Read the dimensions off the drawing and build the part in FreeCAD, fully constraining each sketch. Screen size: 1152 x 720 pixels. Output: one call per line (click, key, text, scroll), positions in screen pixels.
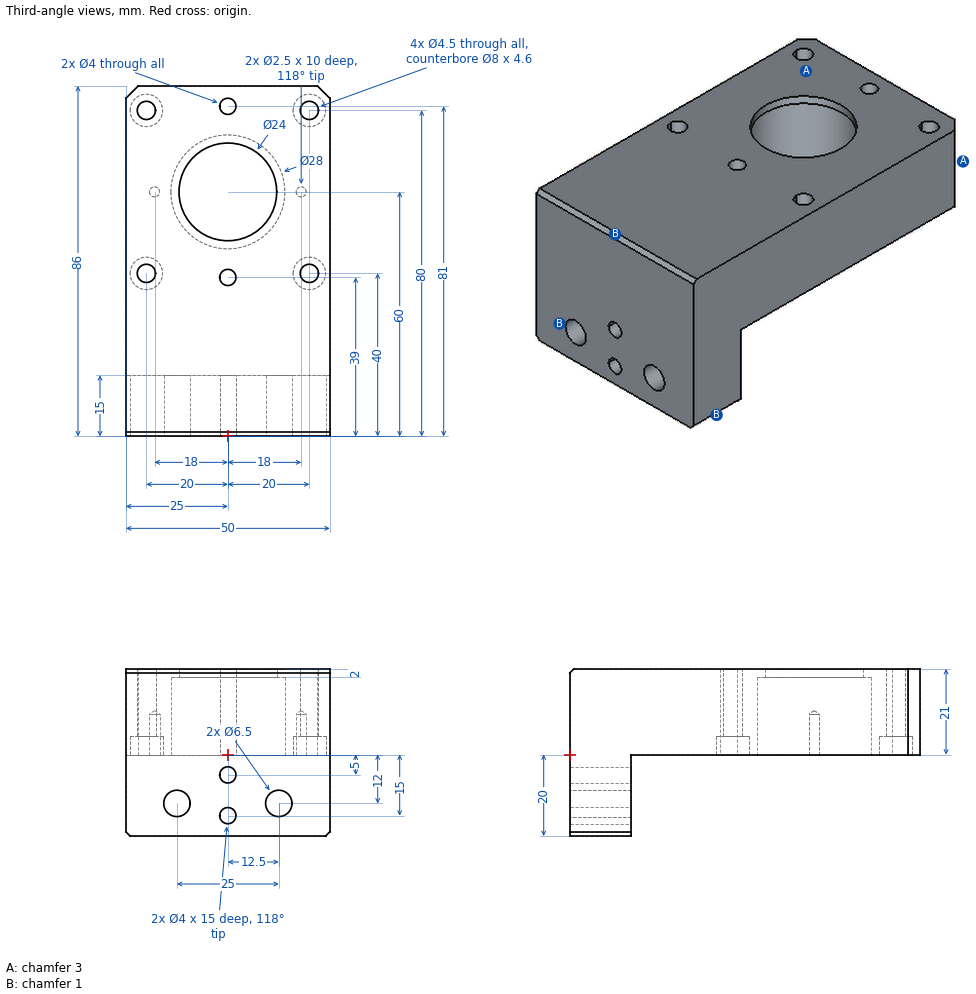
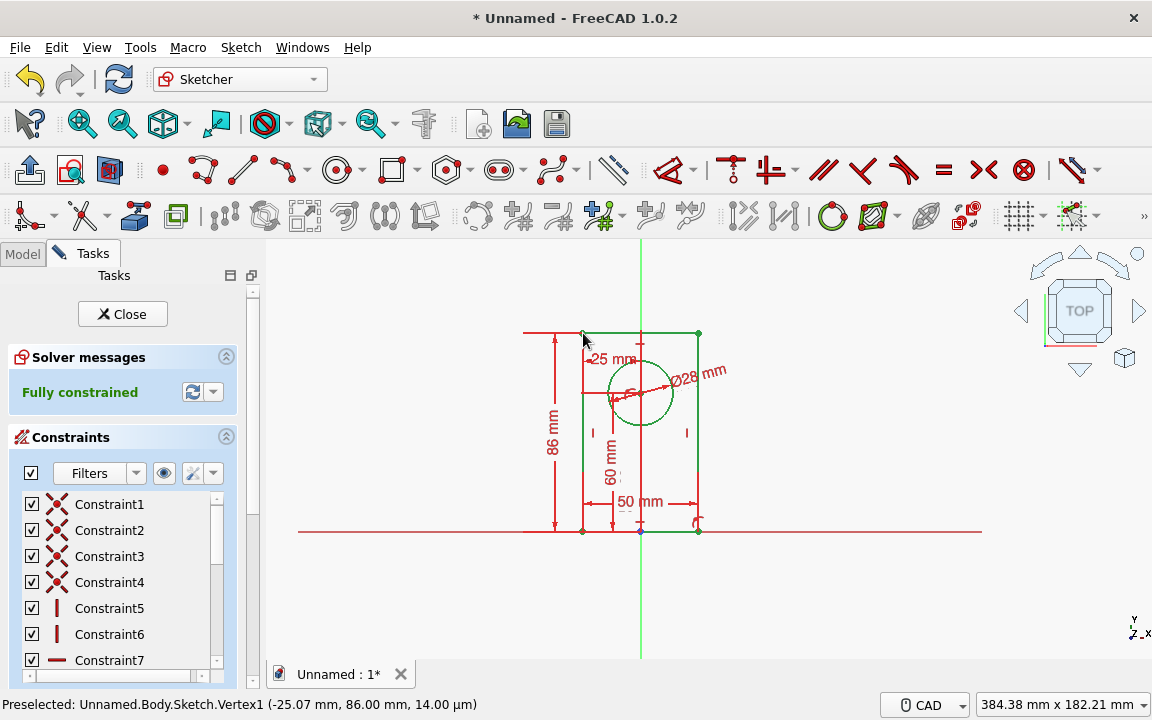
click(123, 314)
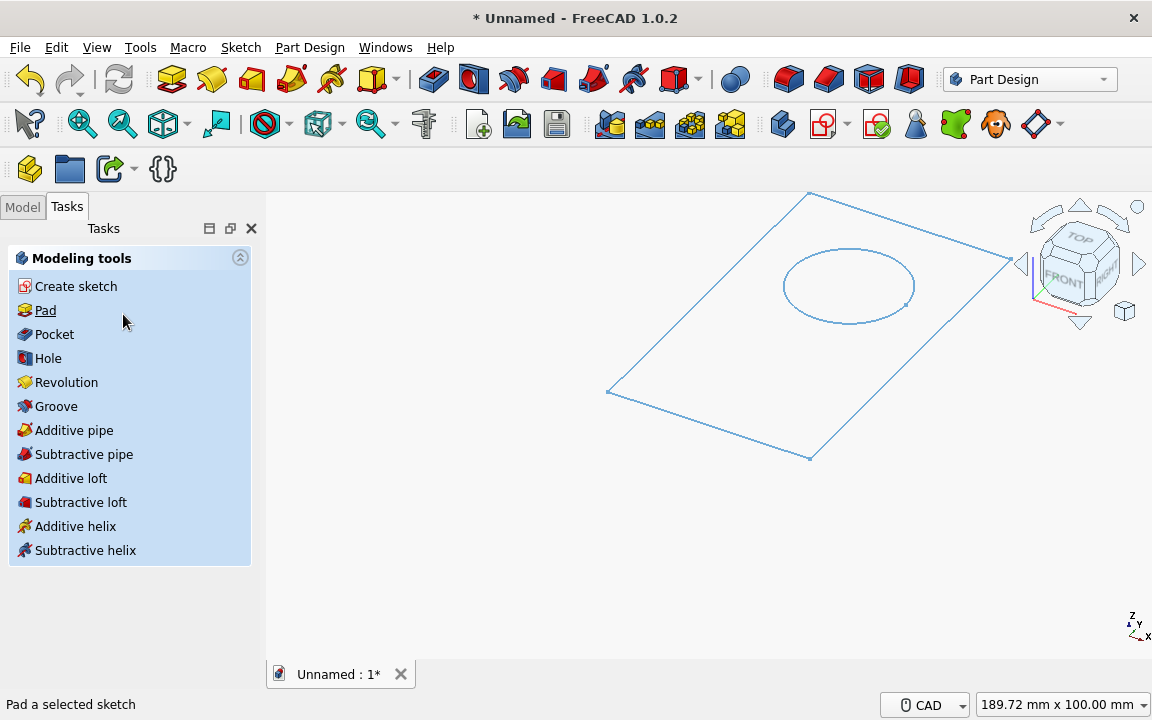
click(172, 80)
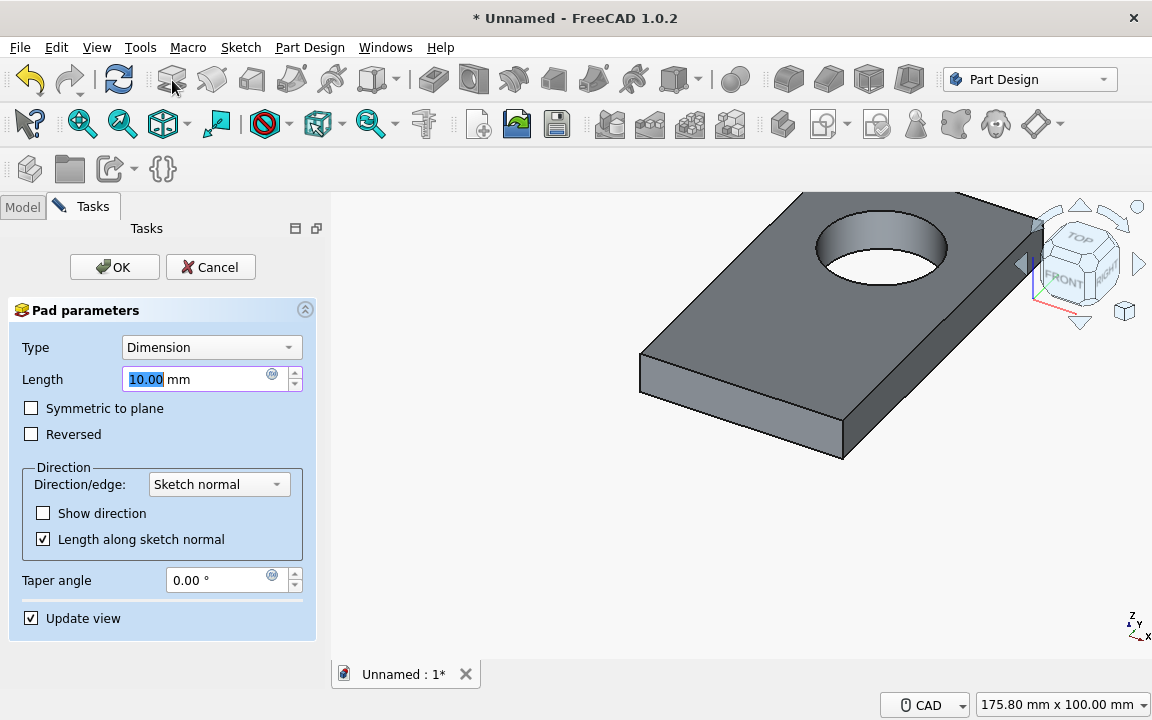
text(21)
key(Tab)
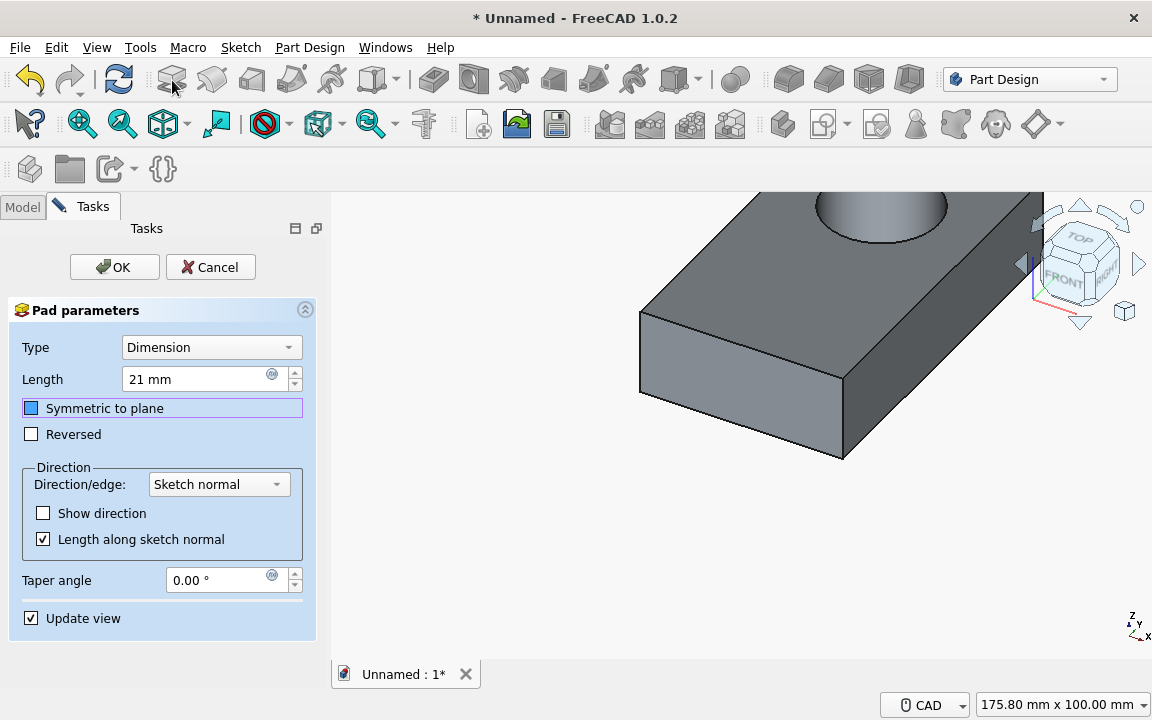
click(115, 267)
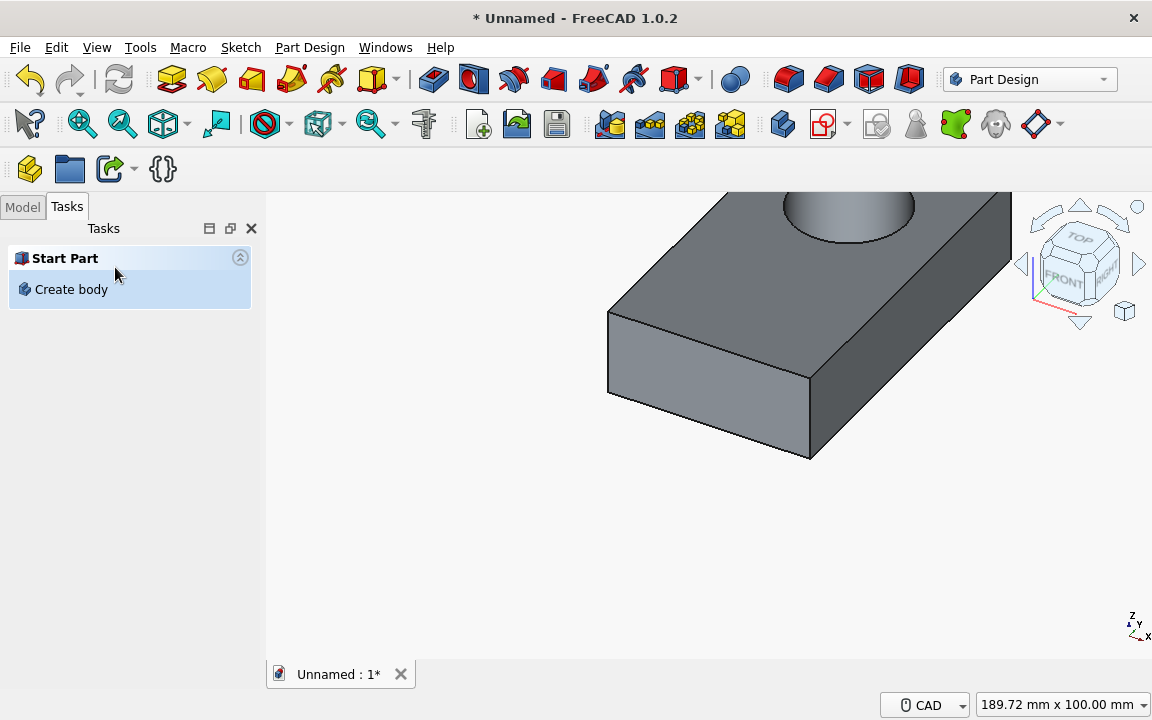
click(84, 124)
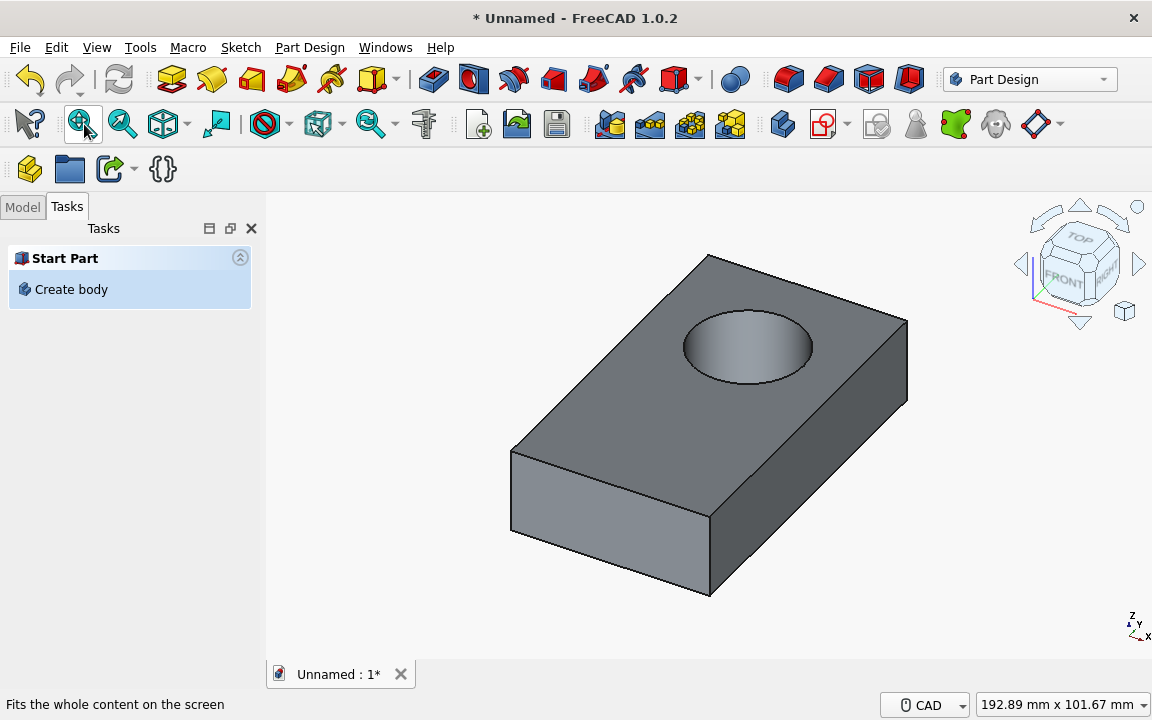
key(5)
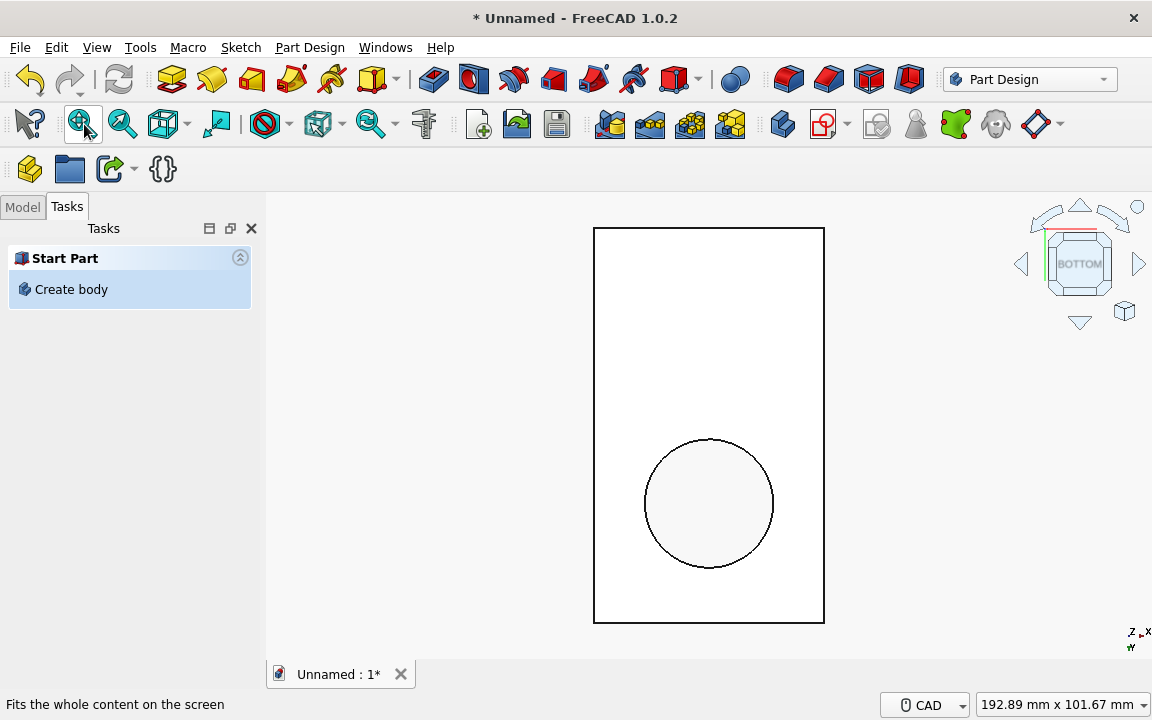
click(709, 312)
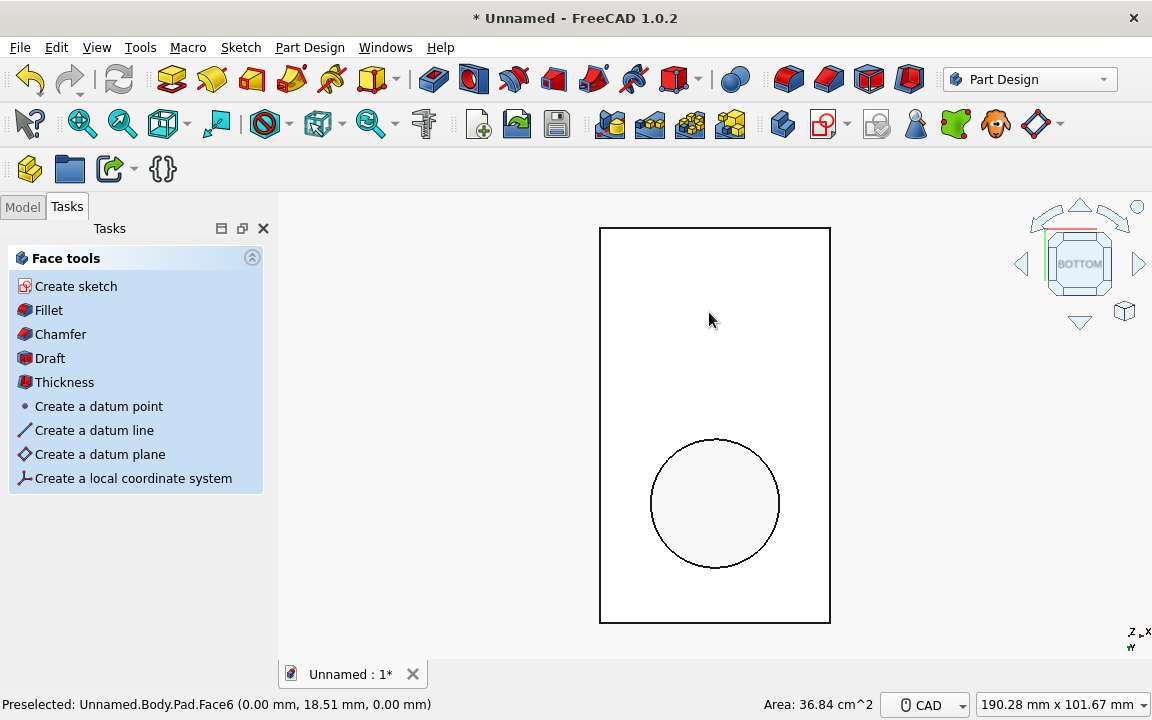
click(824, 124)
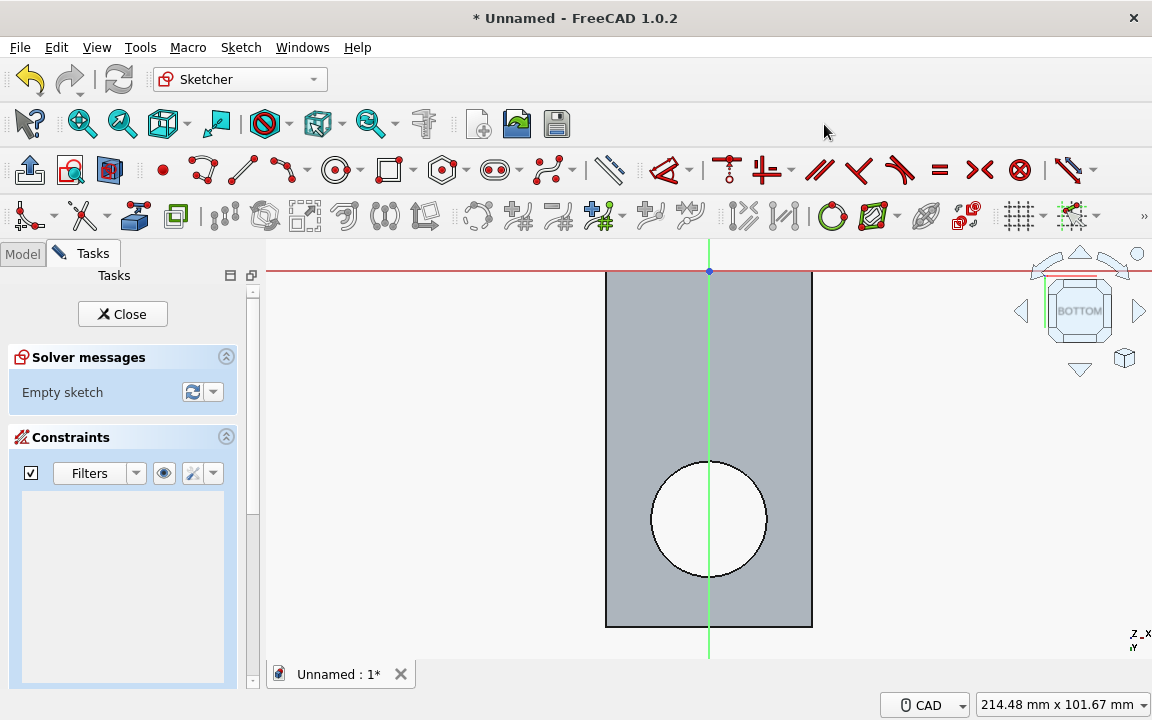
scroll(331, 631, down, 1)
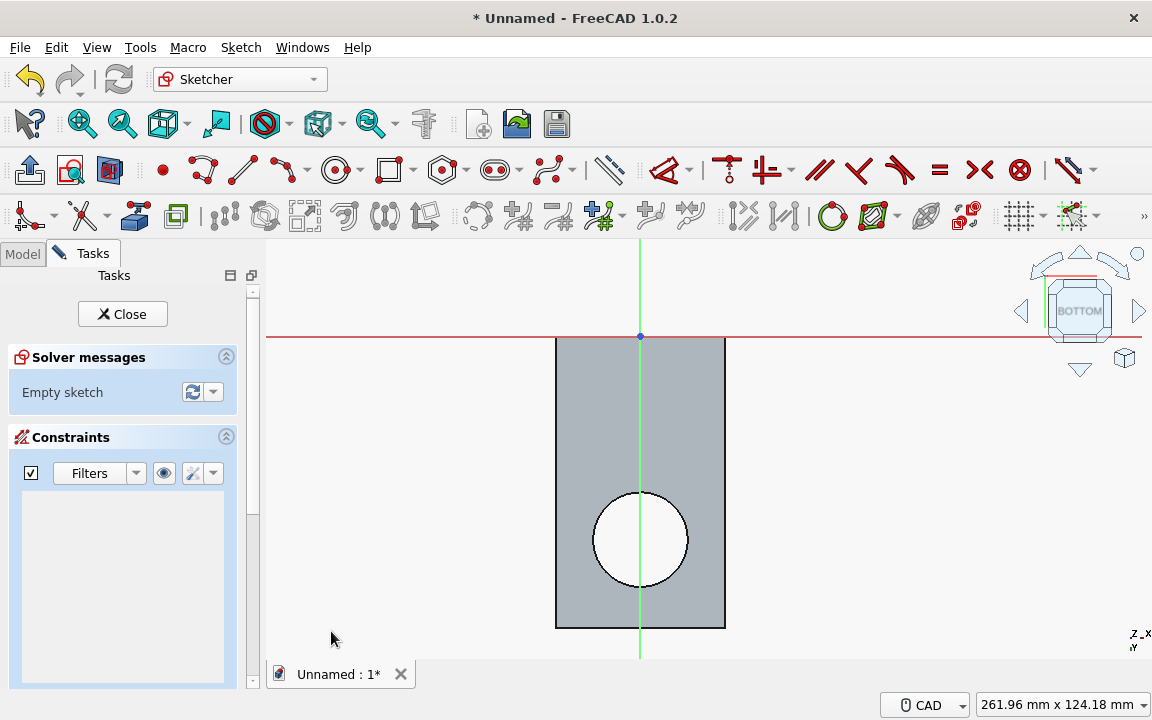
click(336, 170)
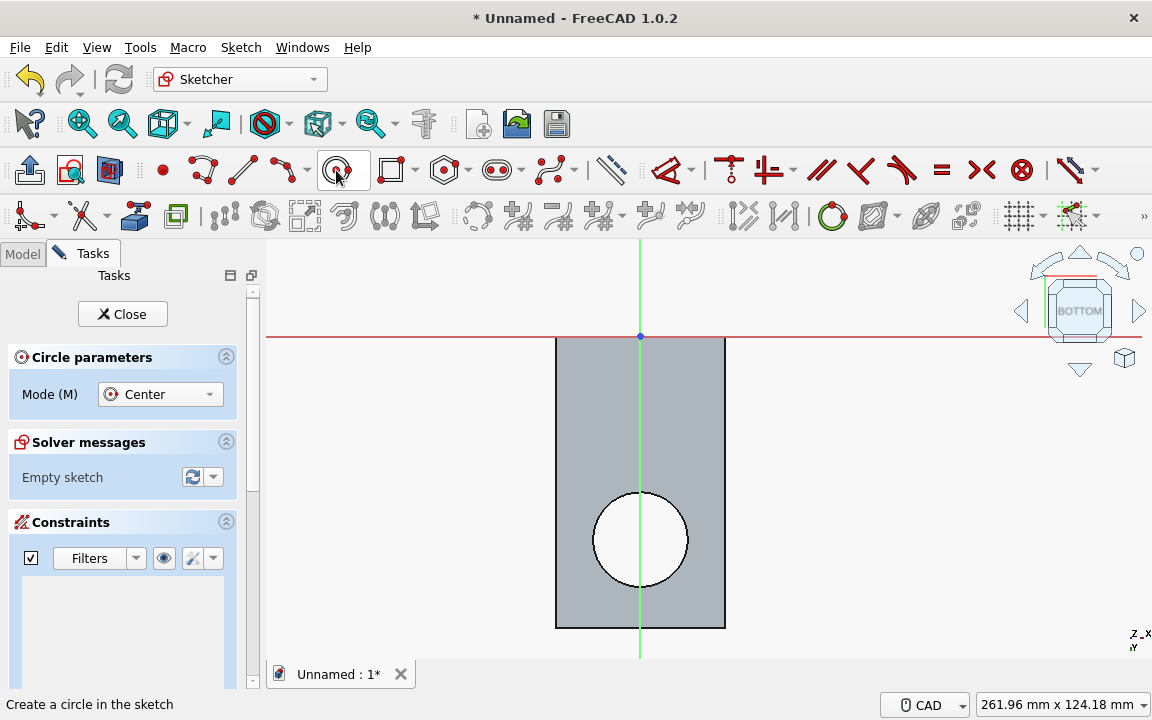
scroll(701, 540, up, 9)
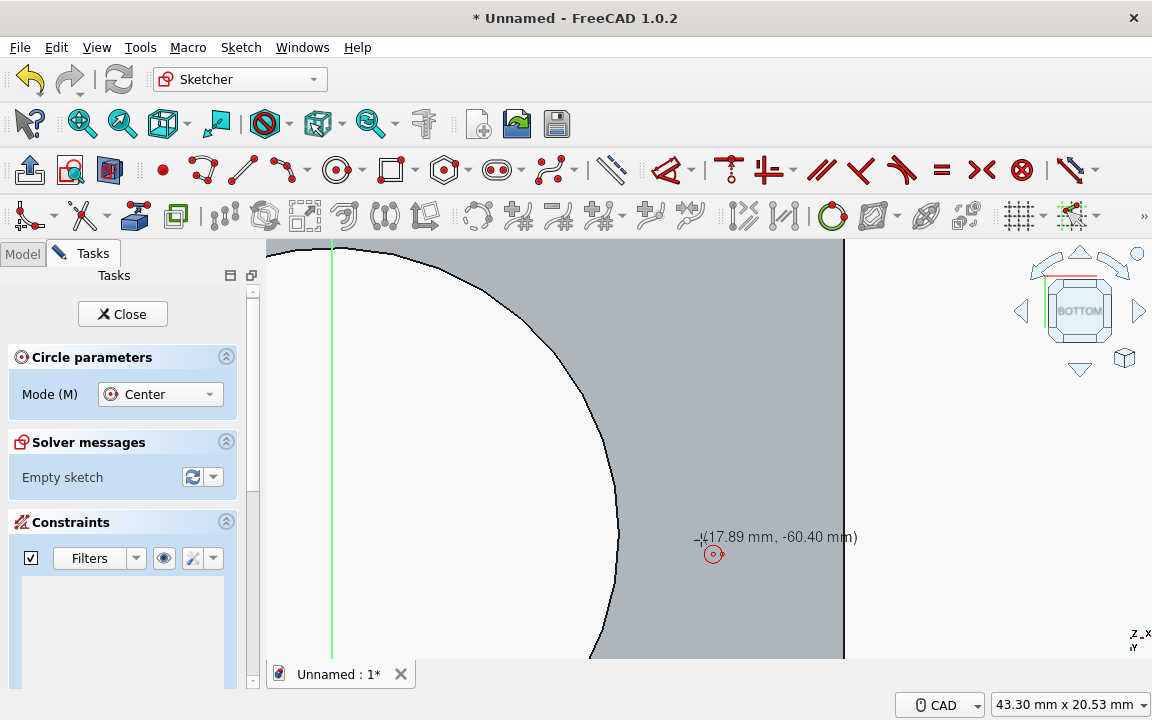
scroll(718, 579, down, 8)